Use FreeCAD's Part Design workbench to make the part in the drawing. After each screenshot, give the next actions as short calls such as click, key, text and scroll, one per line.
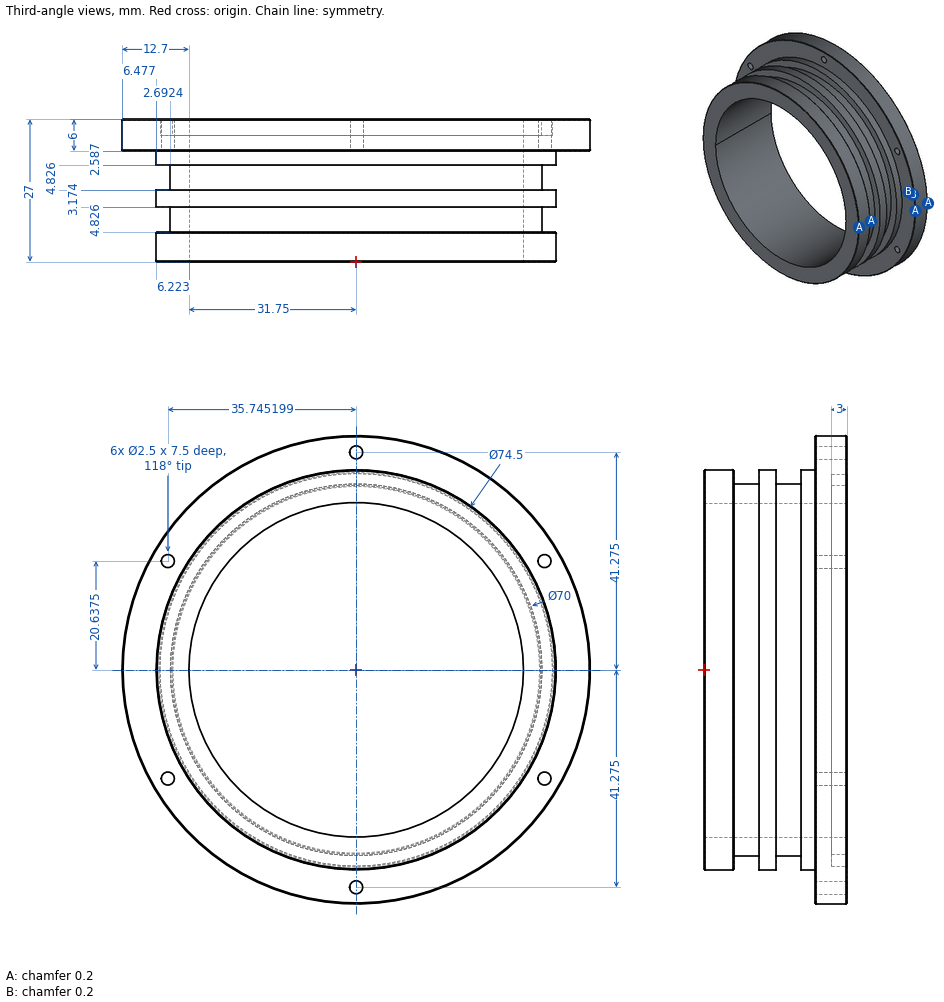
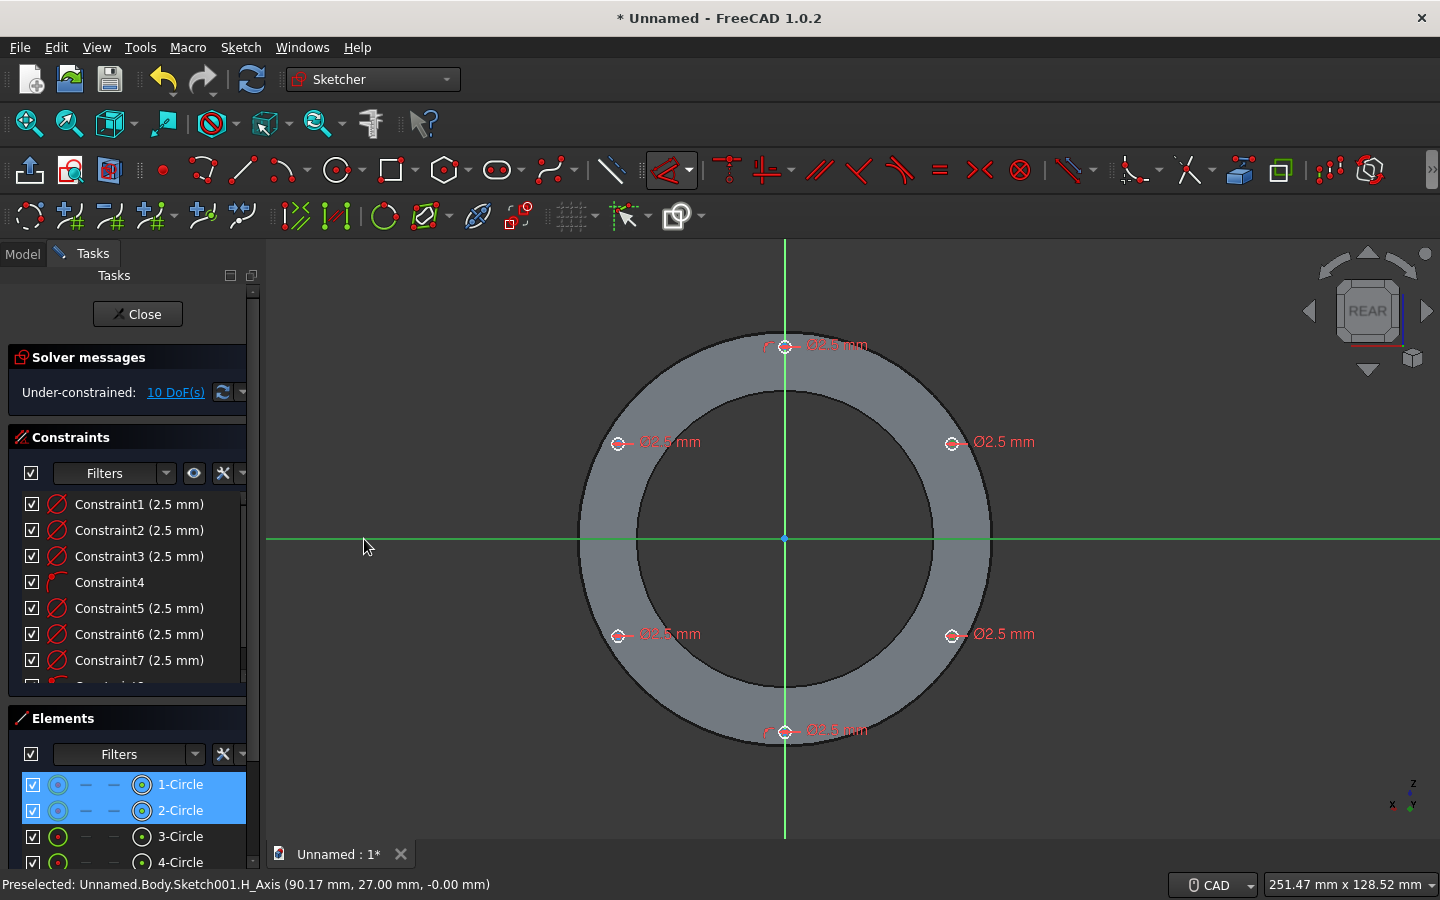
key(s)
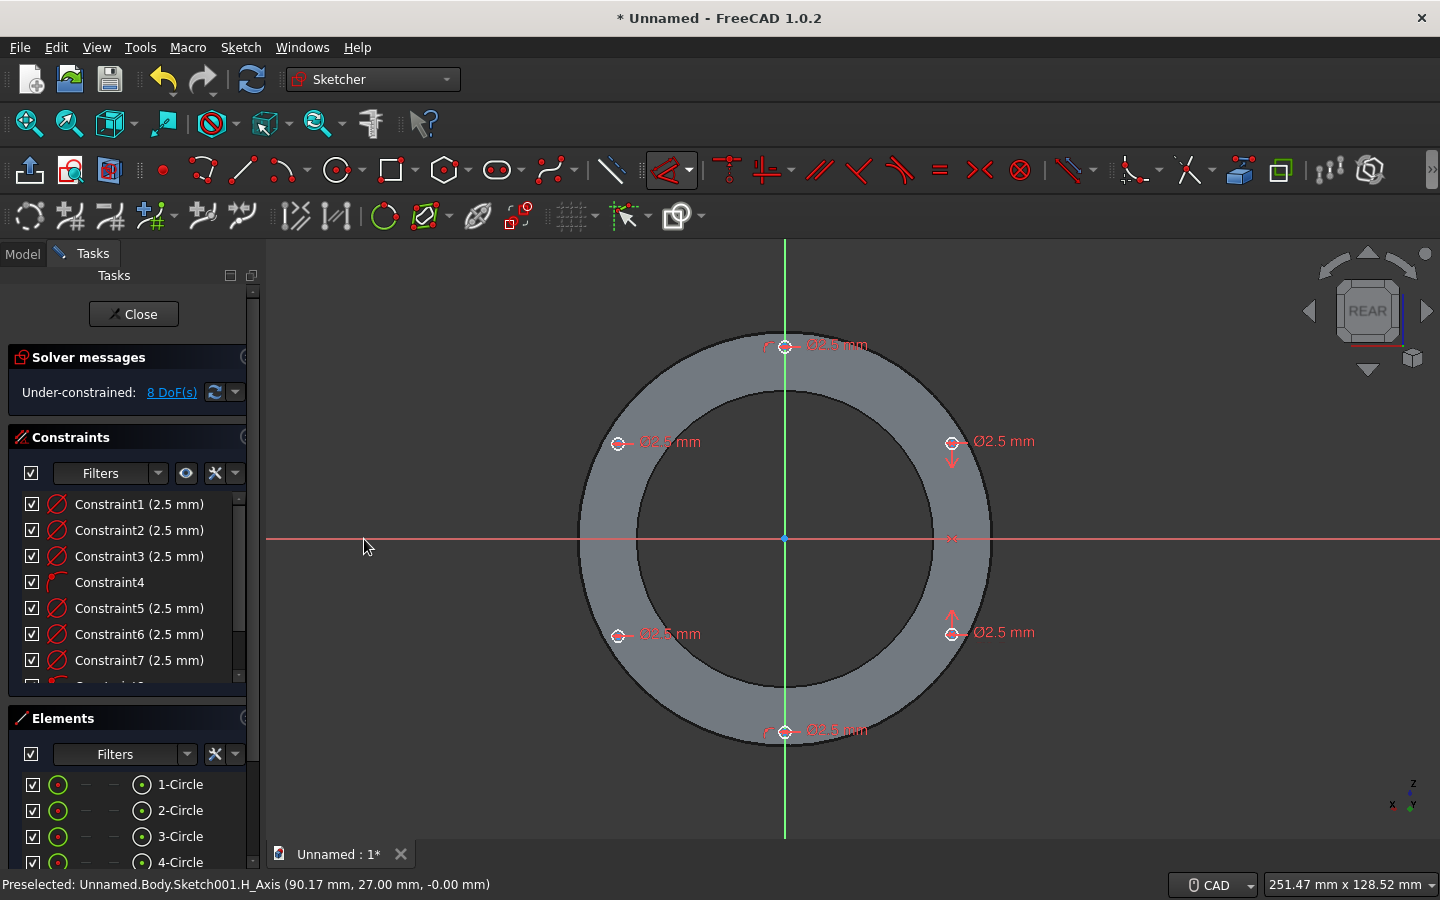
click(952, 635)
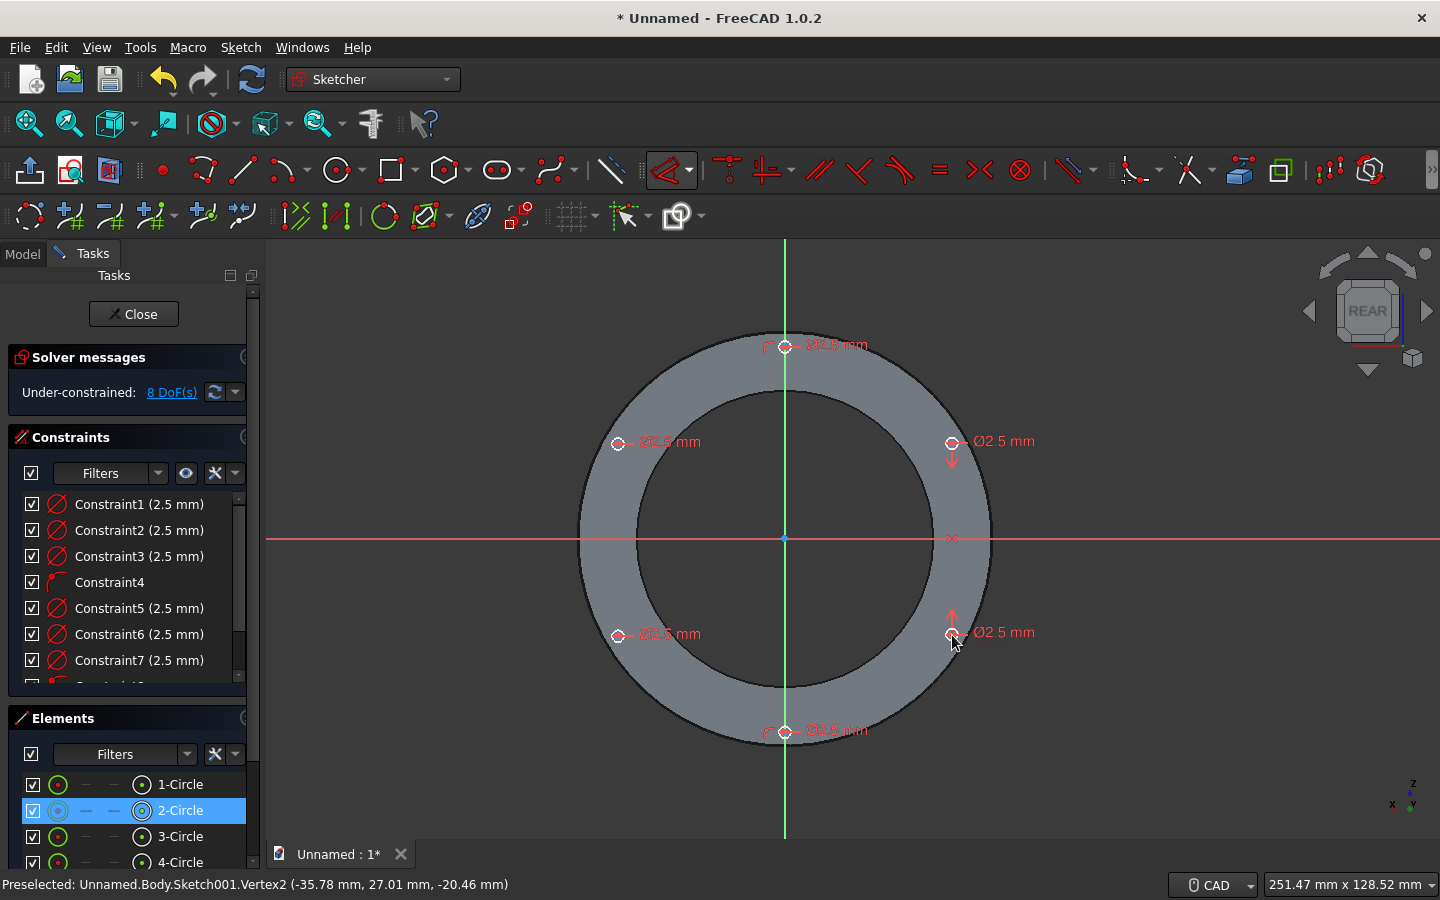
click(618, 636)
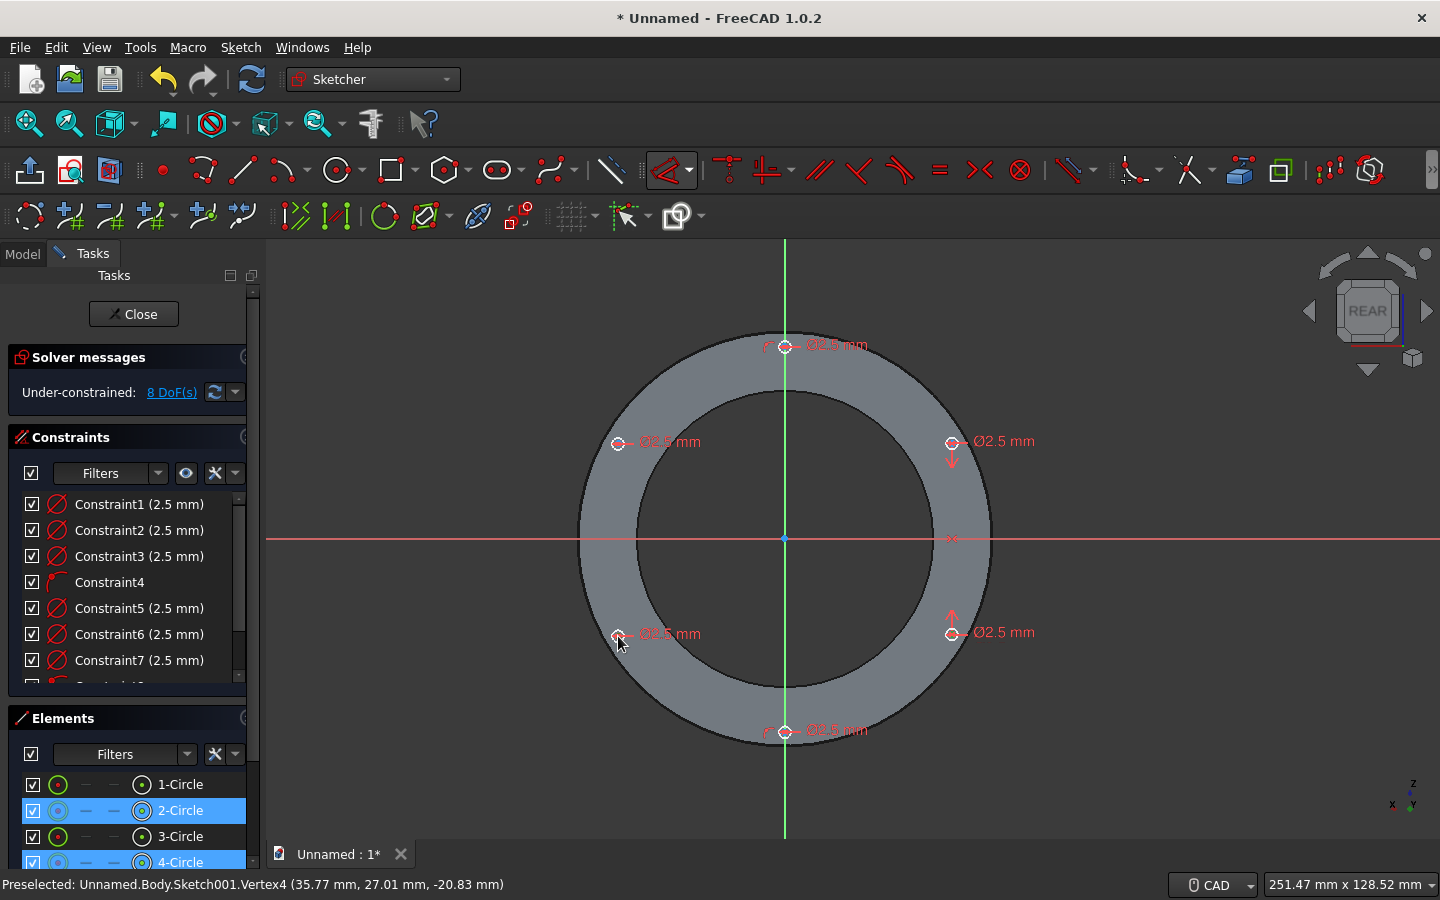
click(785, 772)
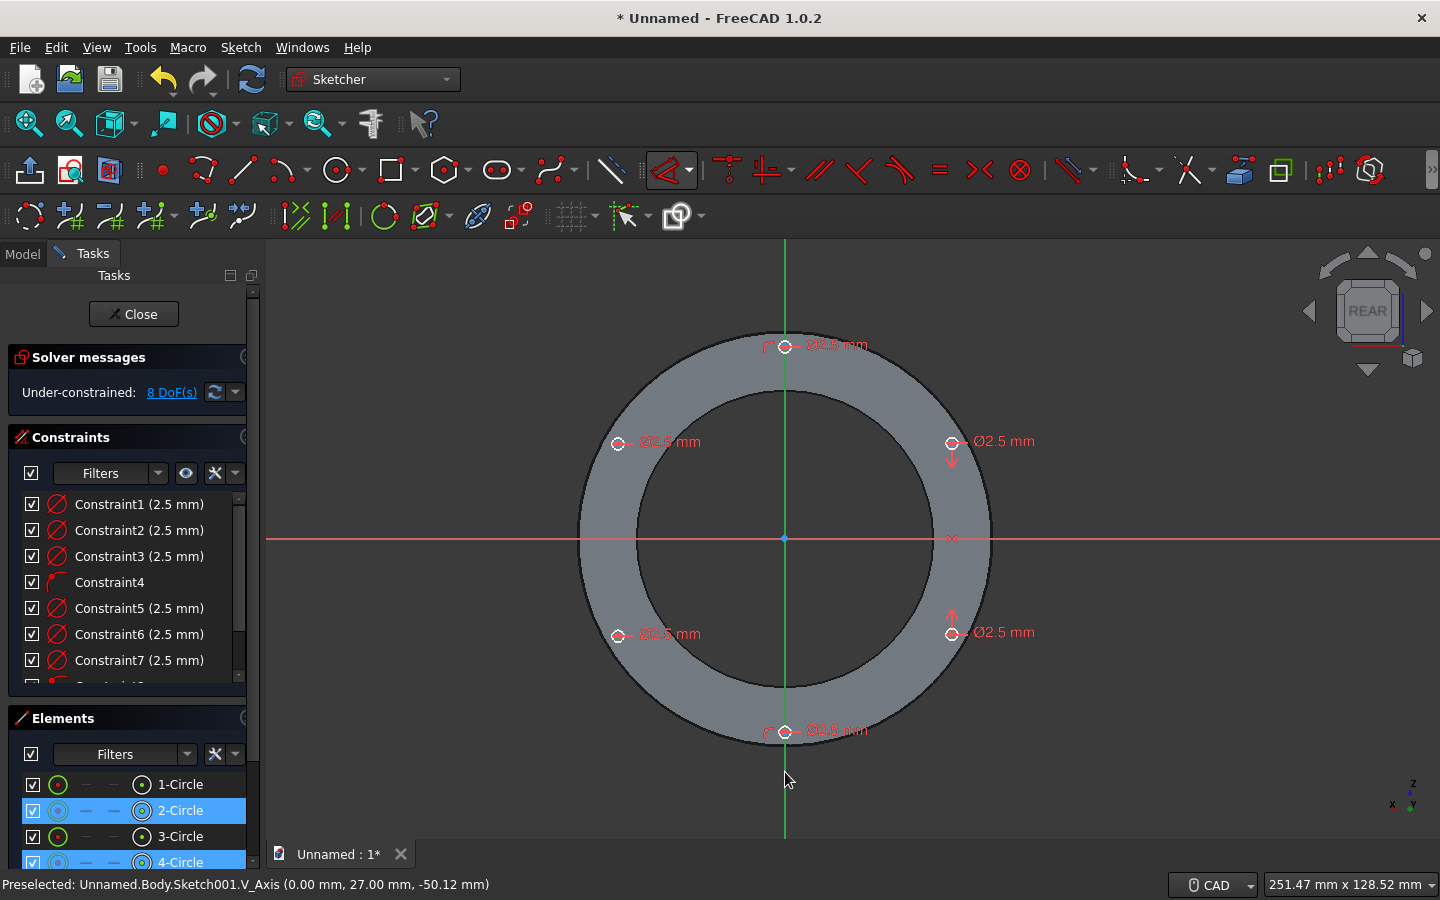
key(s)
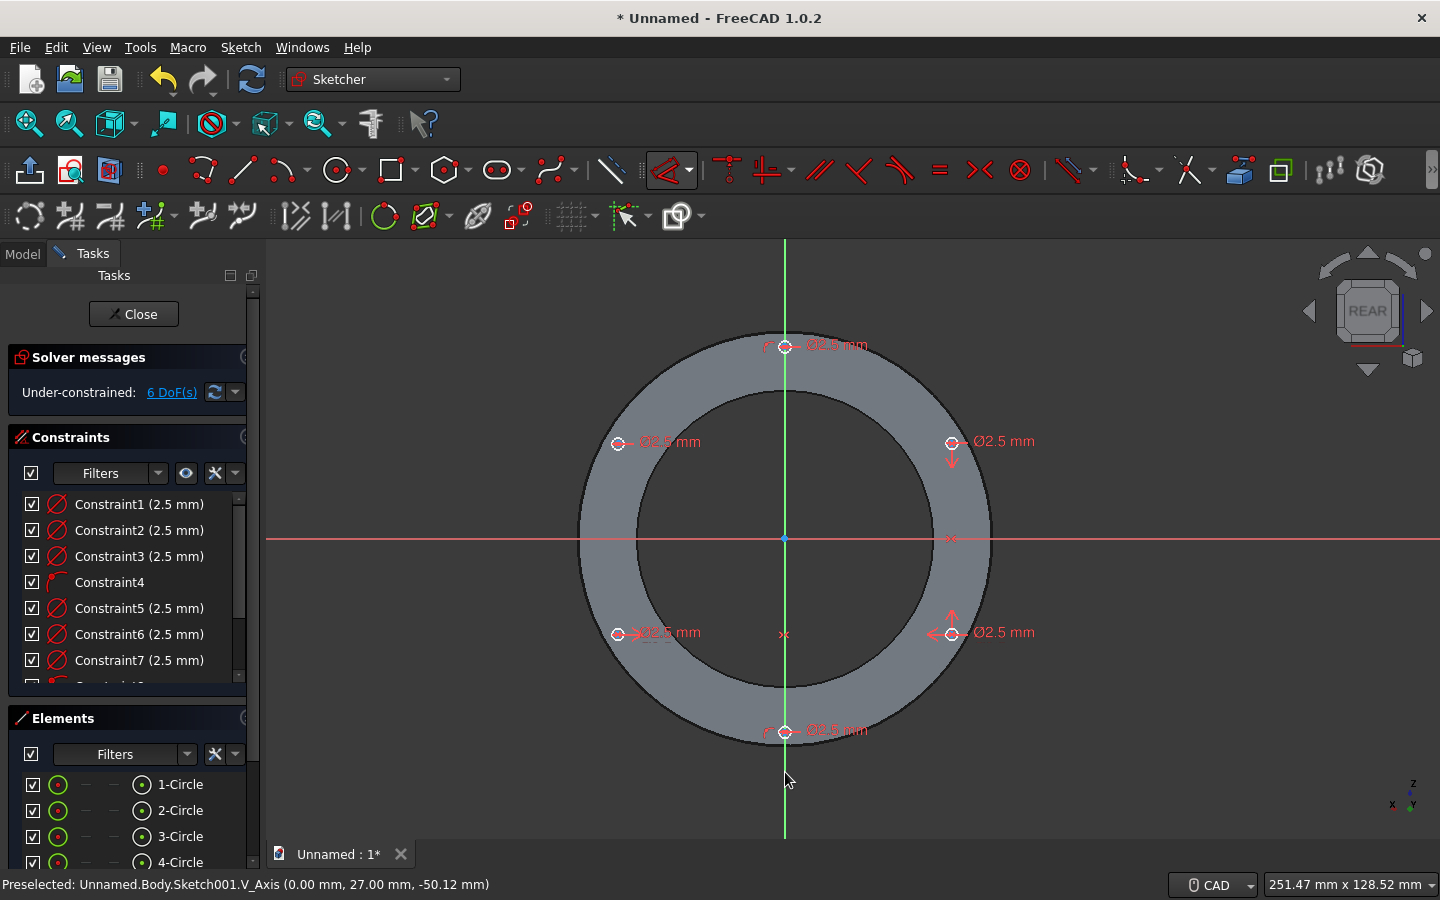
click(952, 443)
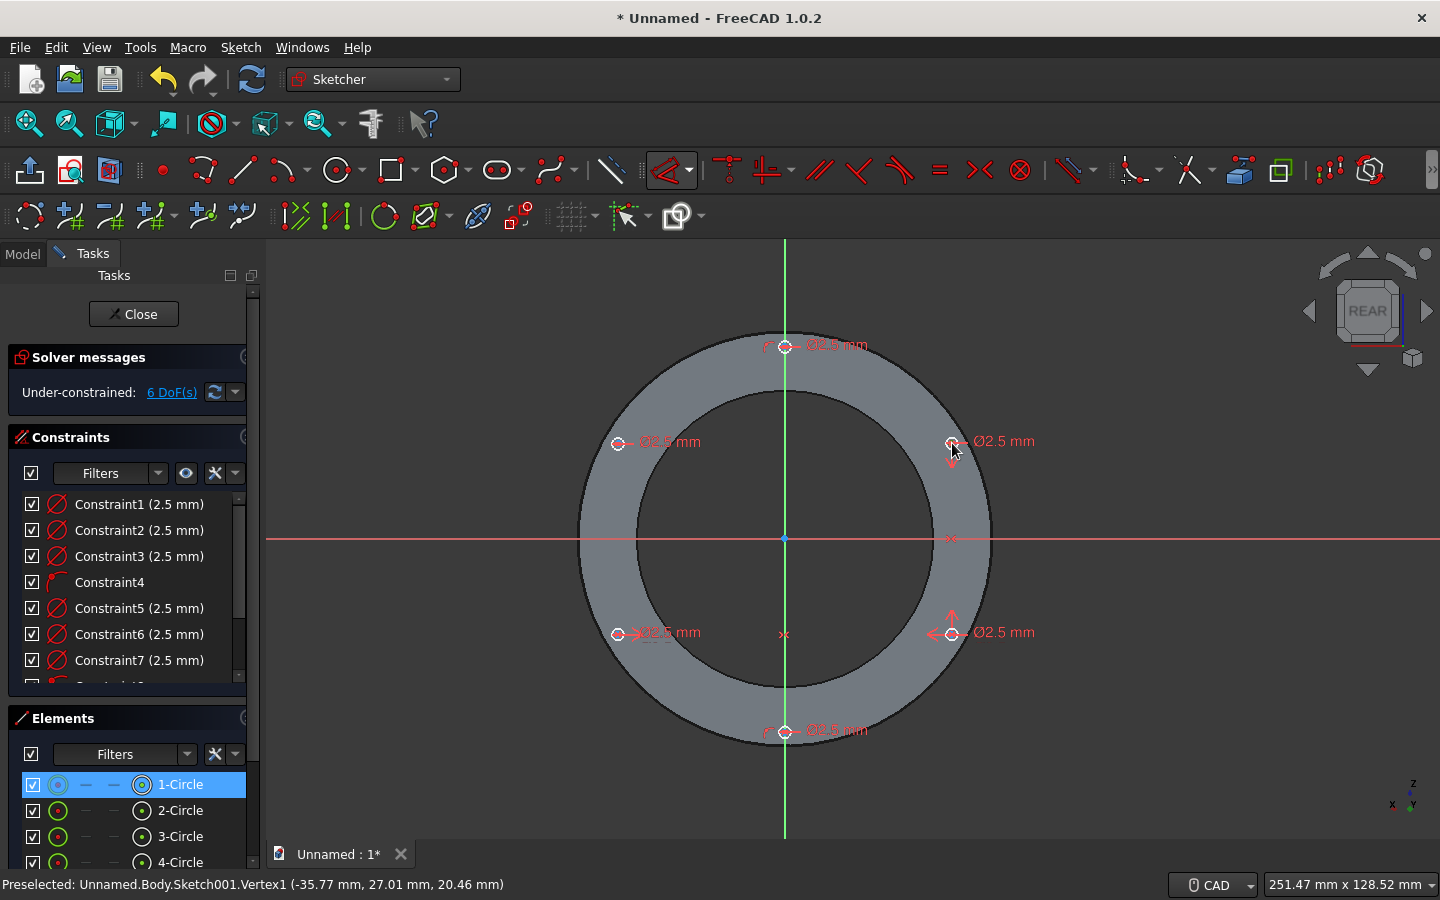
click(618, 444)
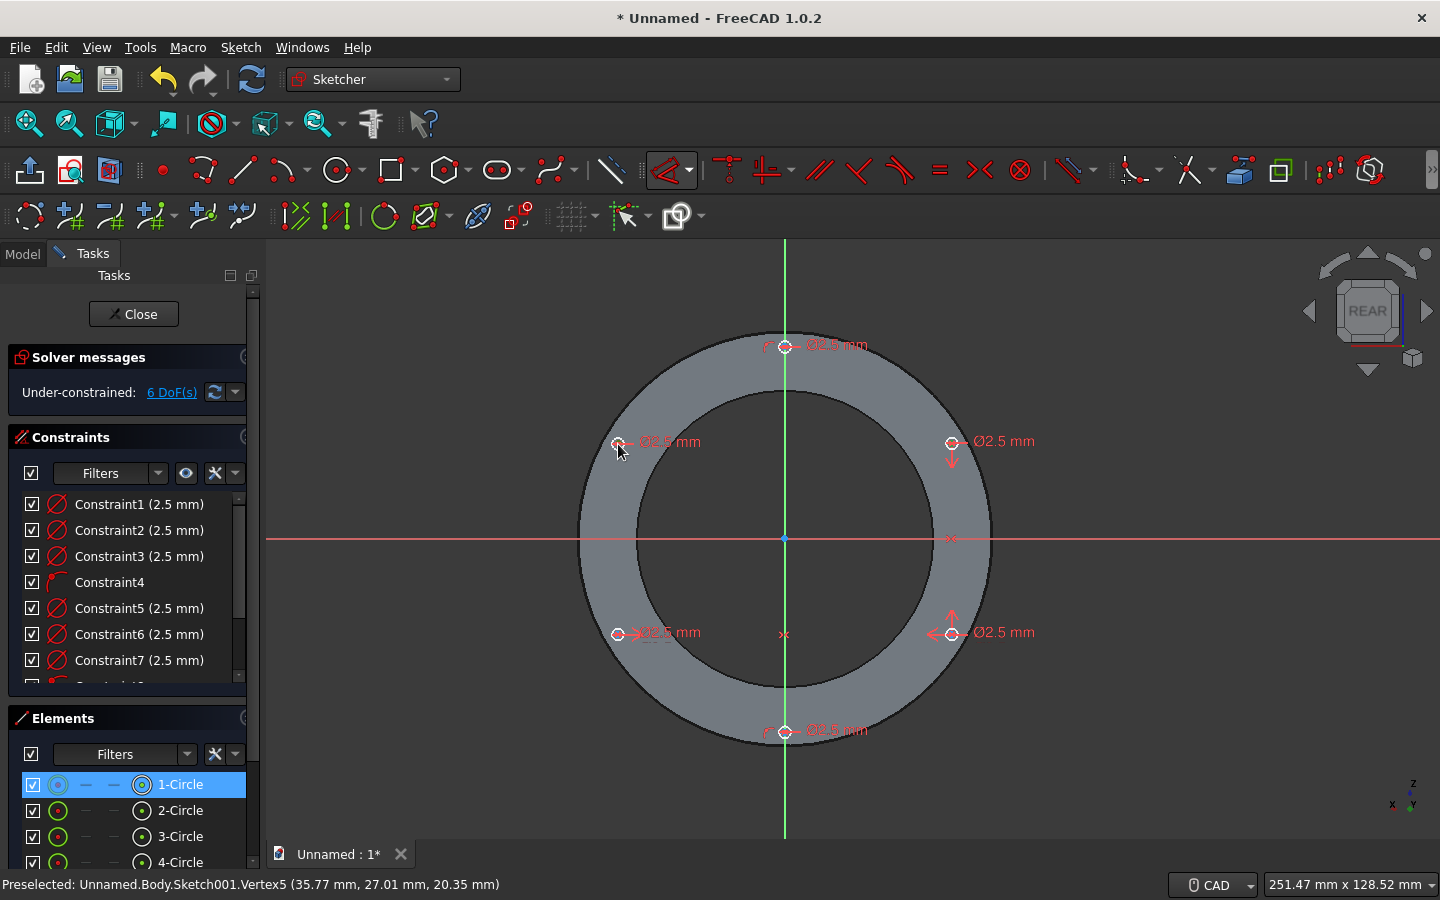
click(785, 772)